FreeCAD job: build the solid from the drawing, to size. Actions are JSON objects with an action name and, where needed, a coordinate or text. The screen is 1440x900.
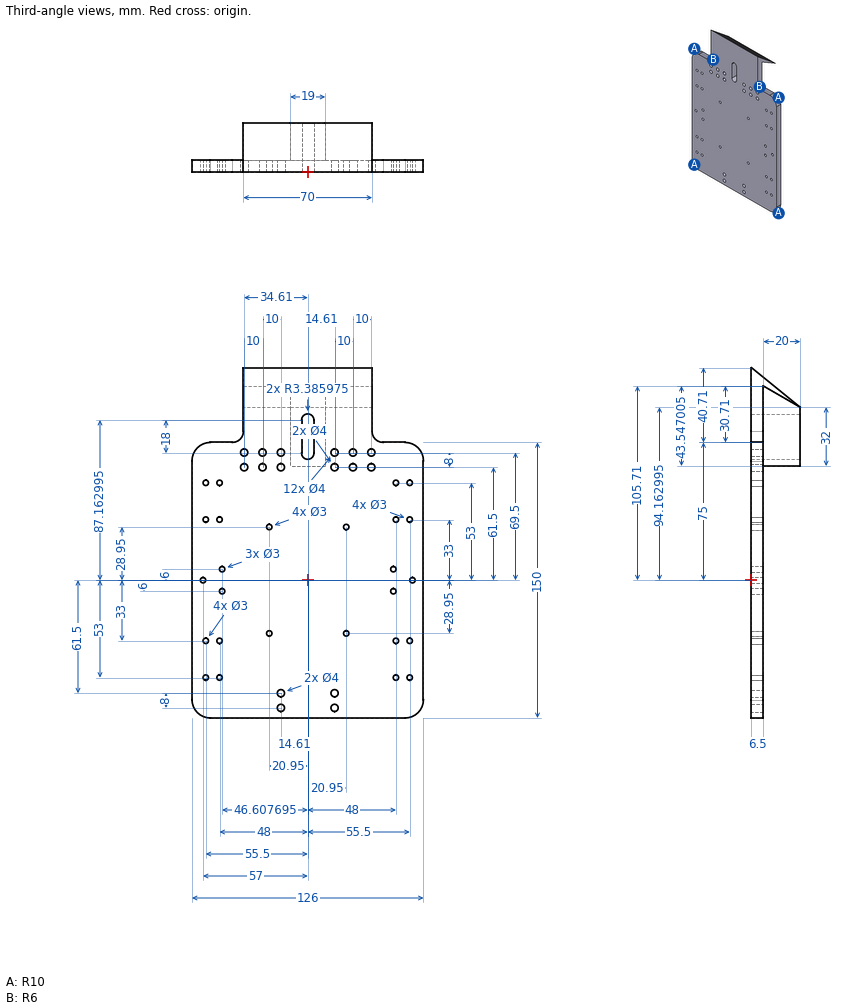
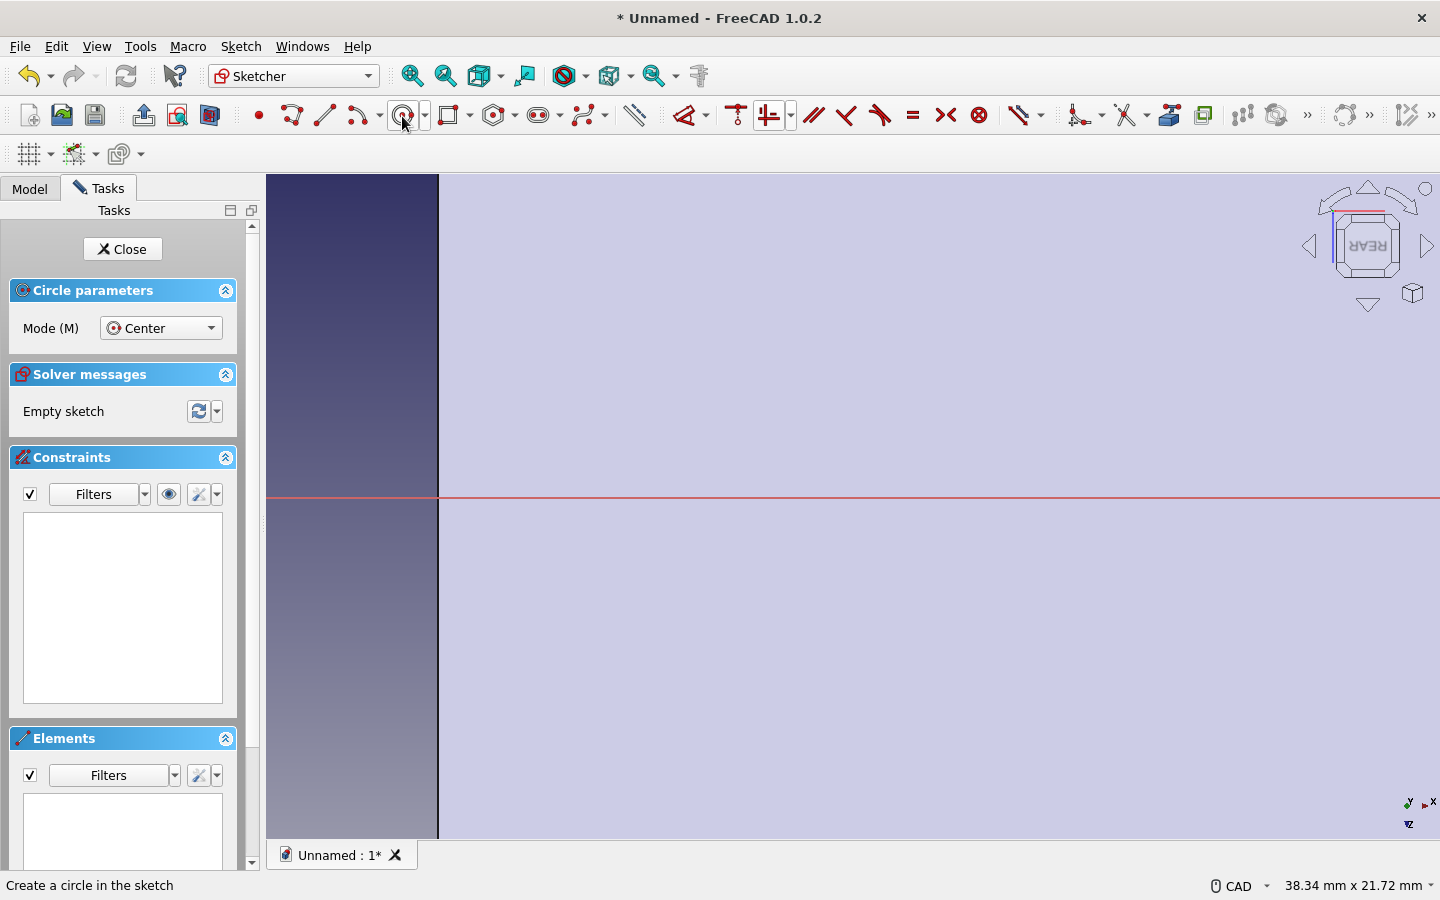
{"action": "left_click", "coordinate": [940, 682]}
{"action": "mouse_move", "coordinate": [972, 650]}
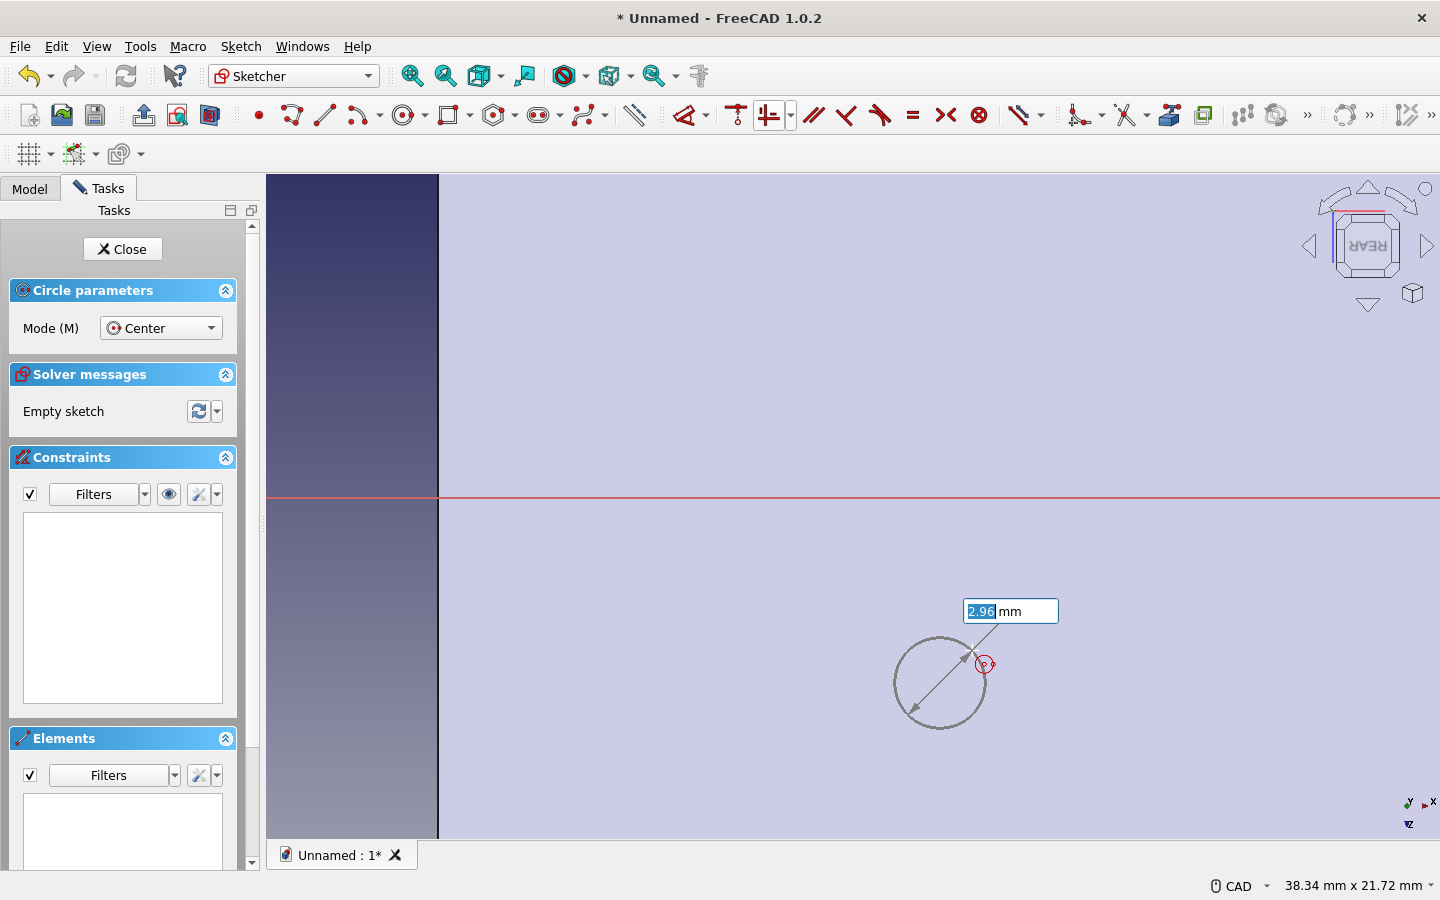
{"action": "type", "text": "3"}
{"action": "key", "text": "Return"}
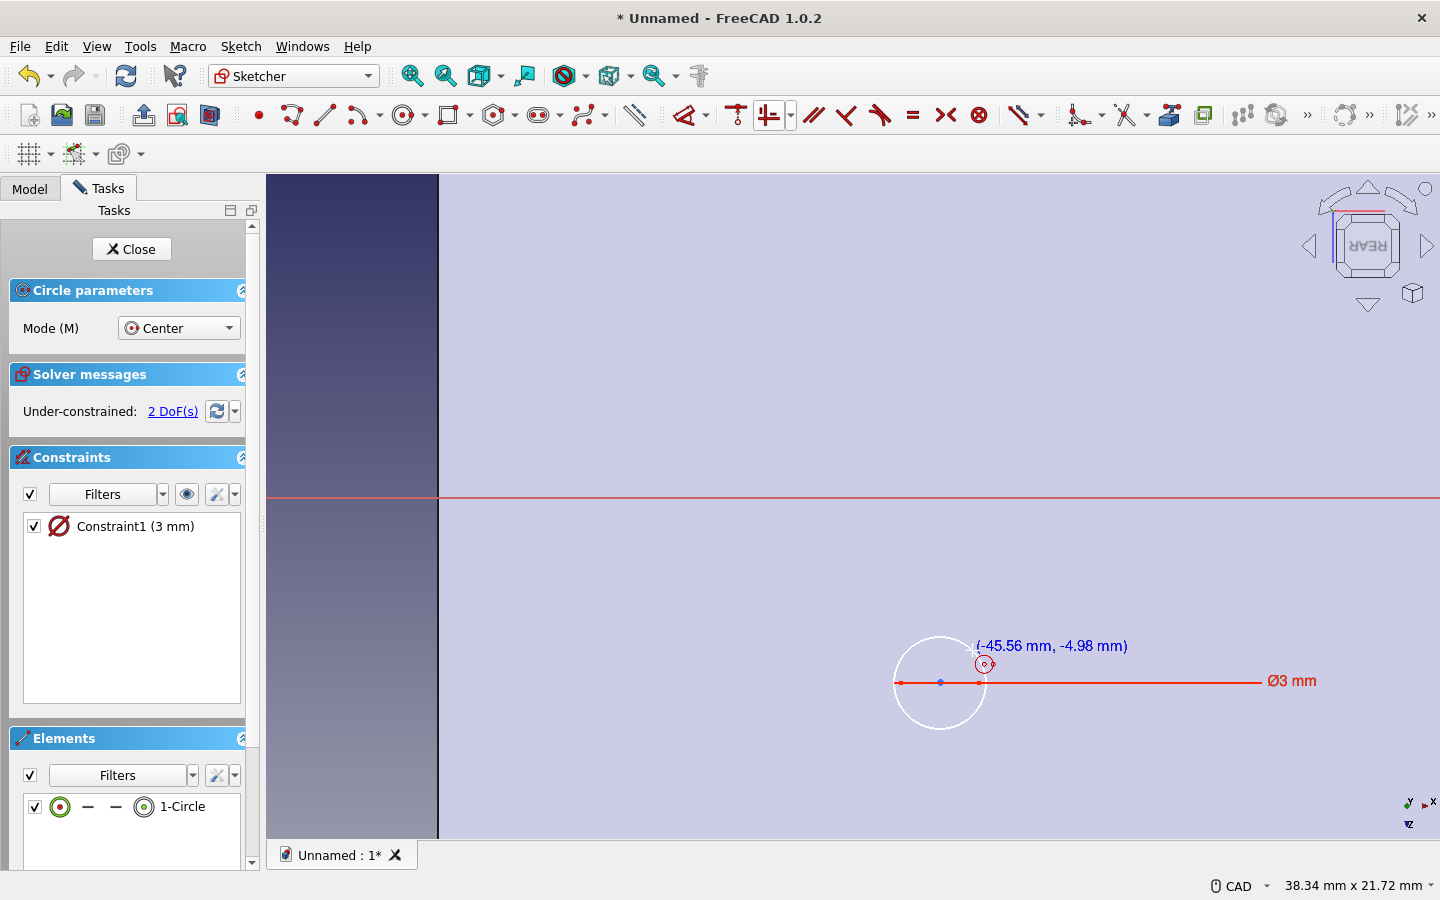
{"action": "left_click", "coordinate": [940, 315]}
{"action": "mouse_move", "coordinate": [972, 282]}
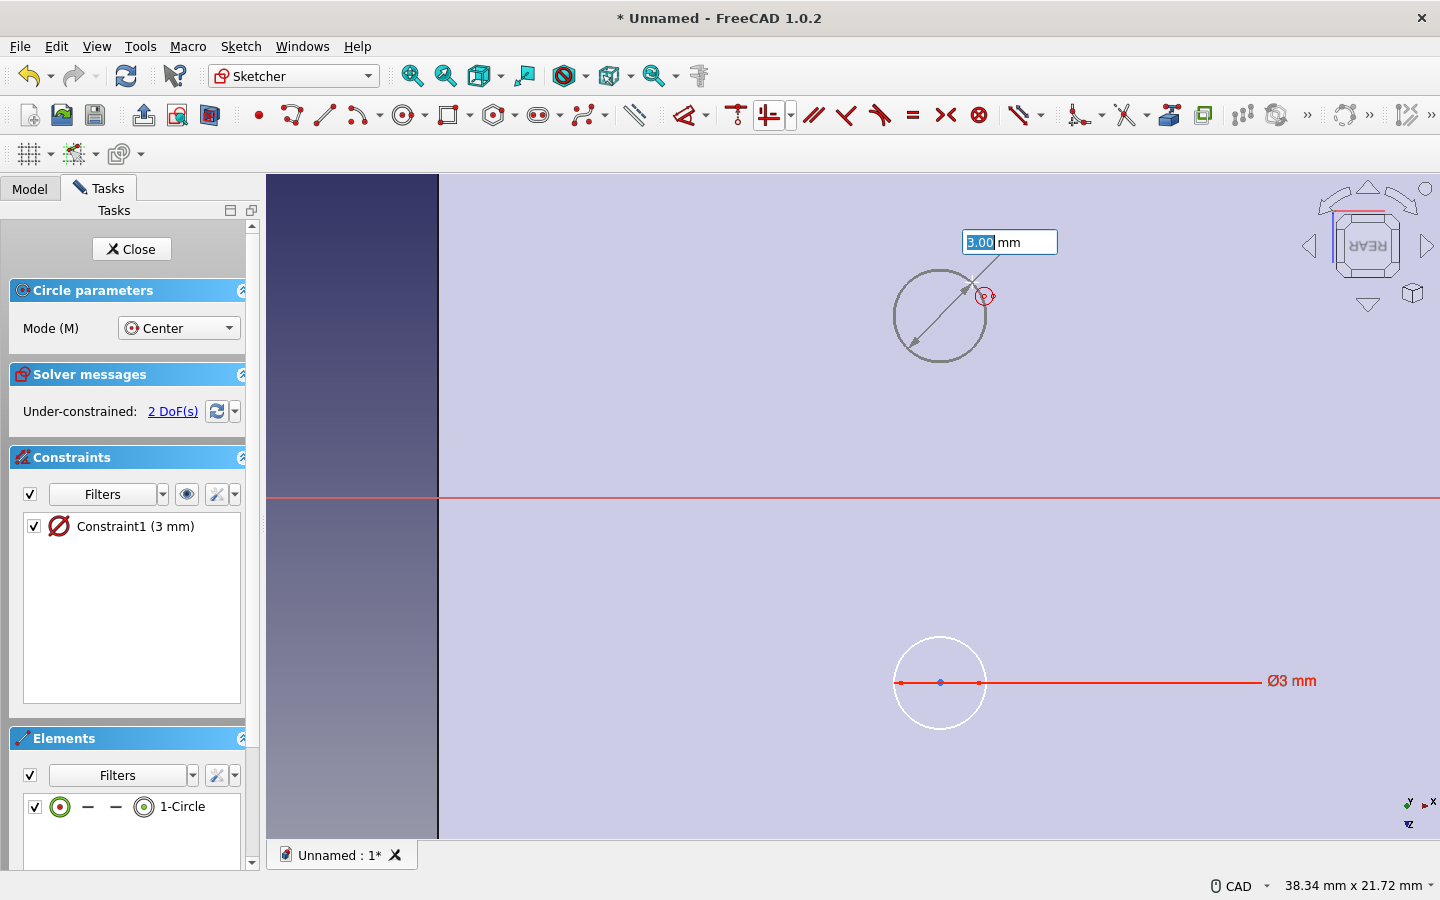
{"action": "type", "text": "3"}
{"action": "key", "text": "Return"}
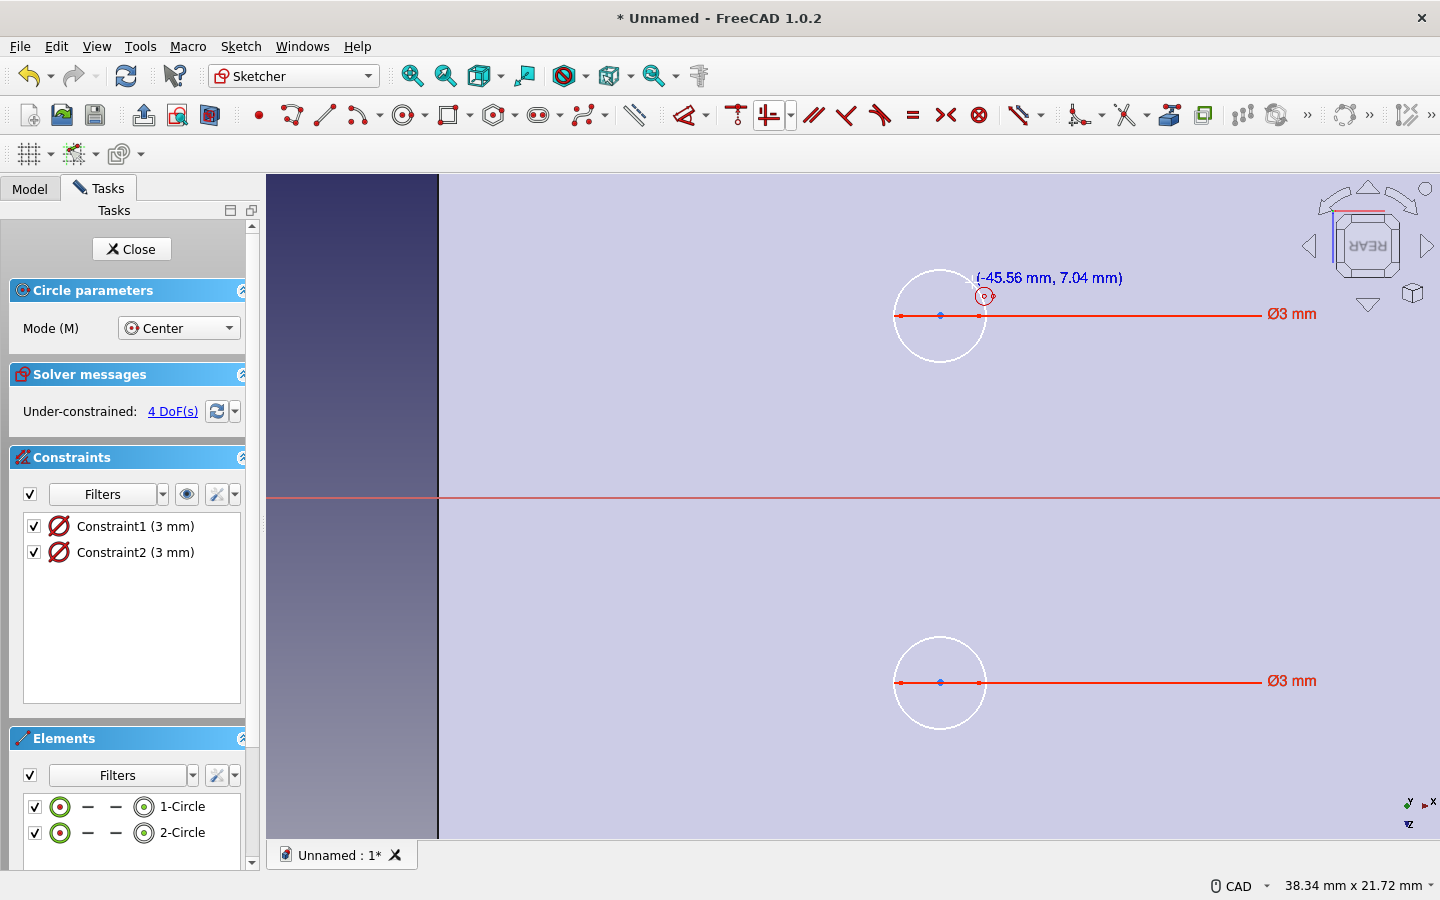
{"action": "left_click", "coordinate": [622, 498]}
{"action": "mouse_move", "coordinate": [654, 466]}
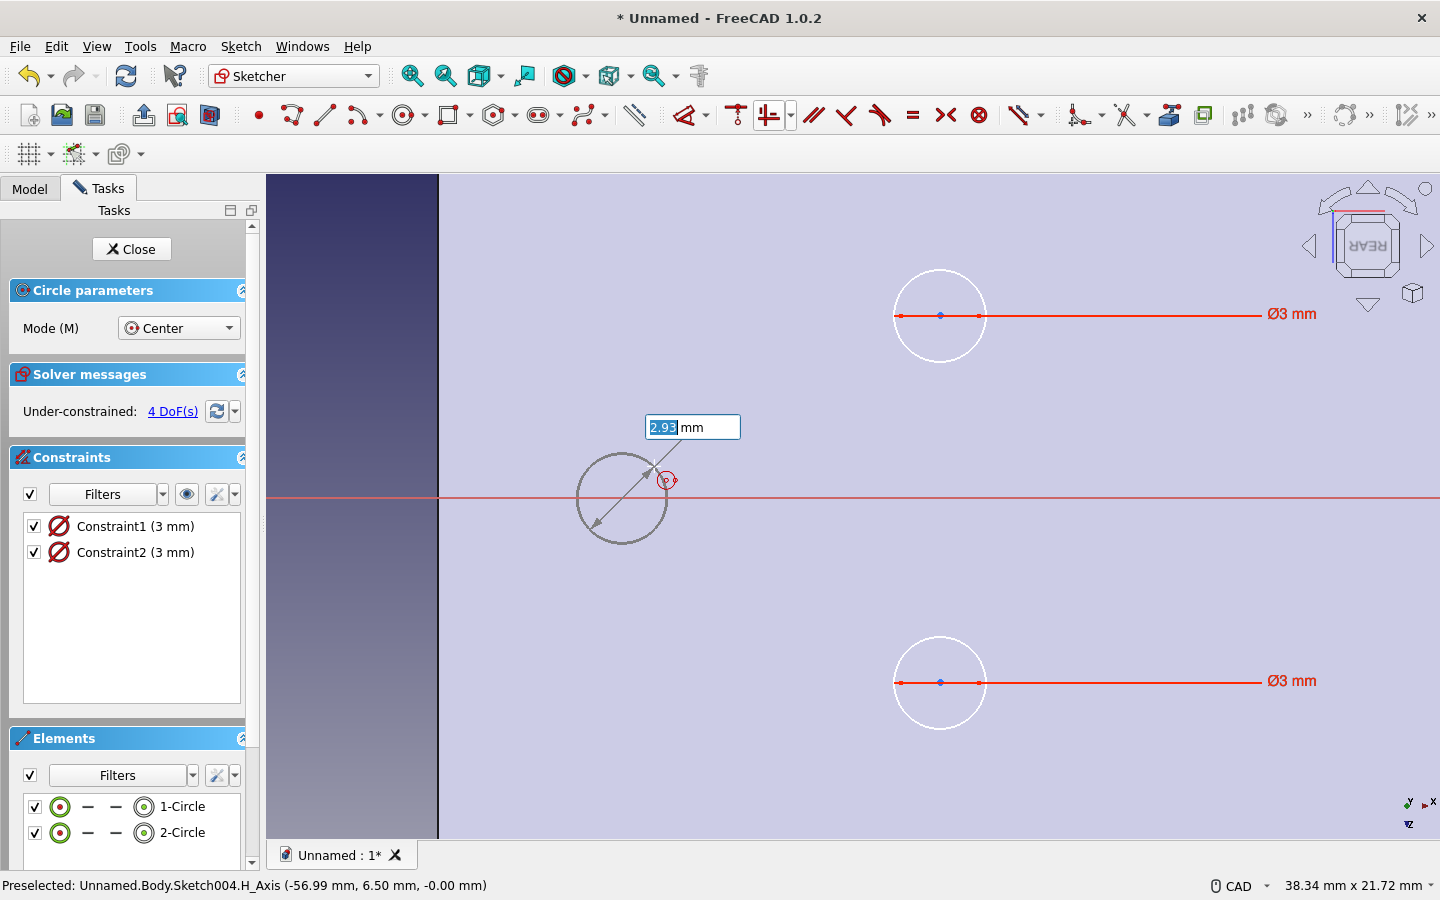
{"action": "type", "text": "3"}
{"action": "key", "text": "Return"}
{"action": "key", "text": "Escape"}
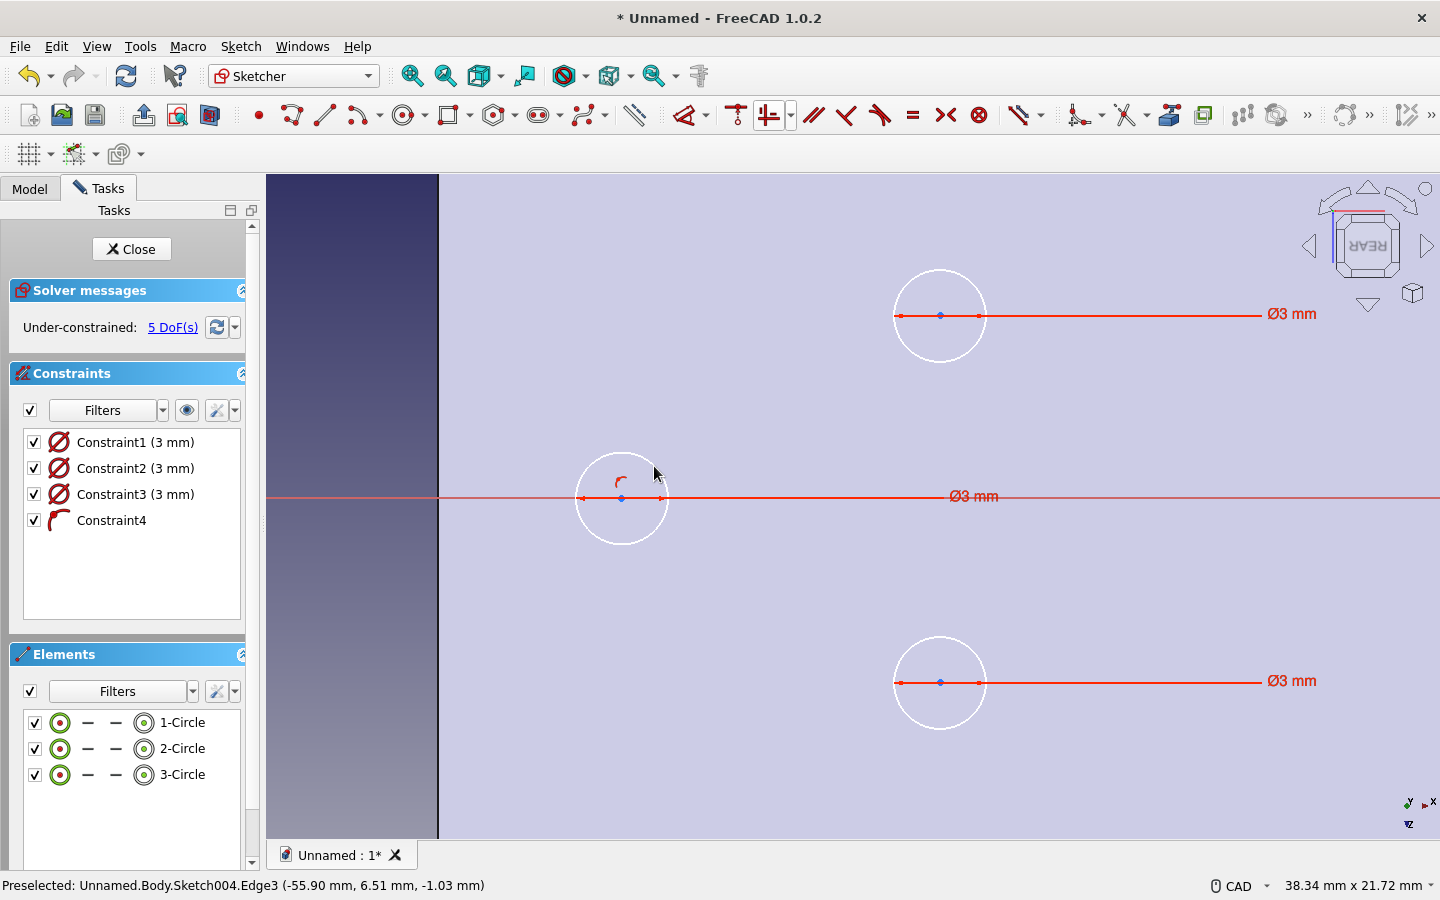
{"action": "left_click", "coordinate": [940, 683]}